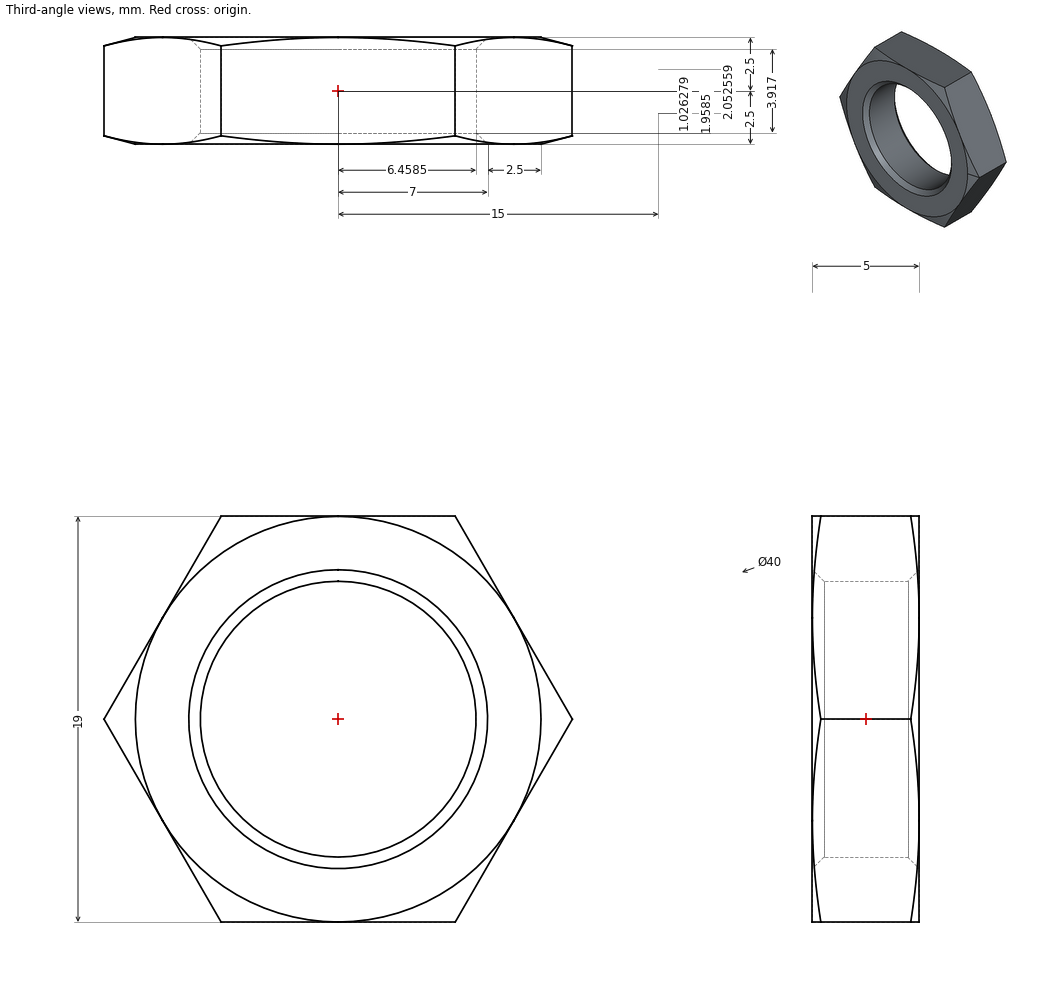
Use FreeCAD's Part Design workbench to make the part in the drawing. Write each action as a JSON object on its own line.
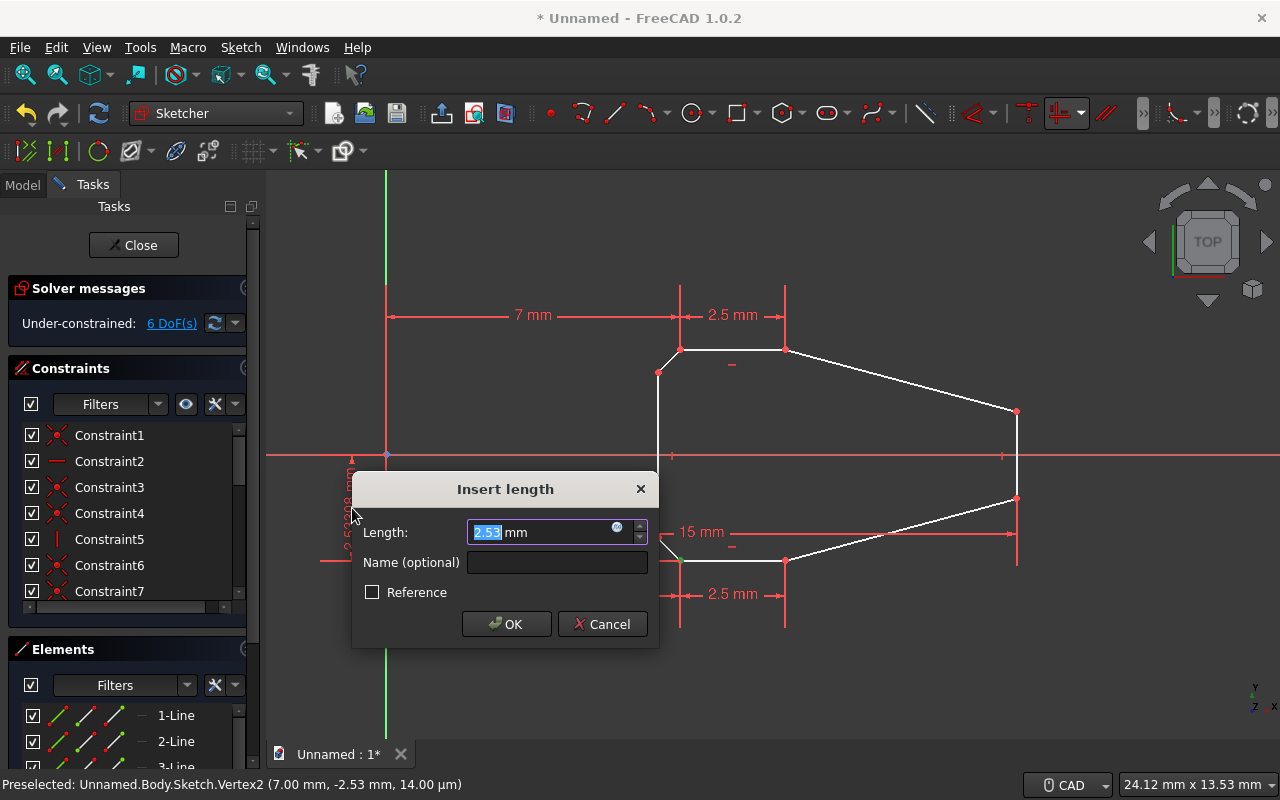
{"action": "type", "text": "2.5"}
{"action": "key", "text": "Return"}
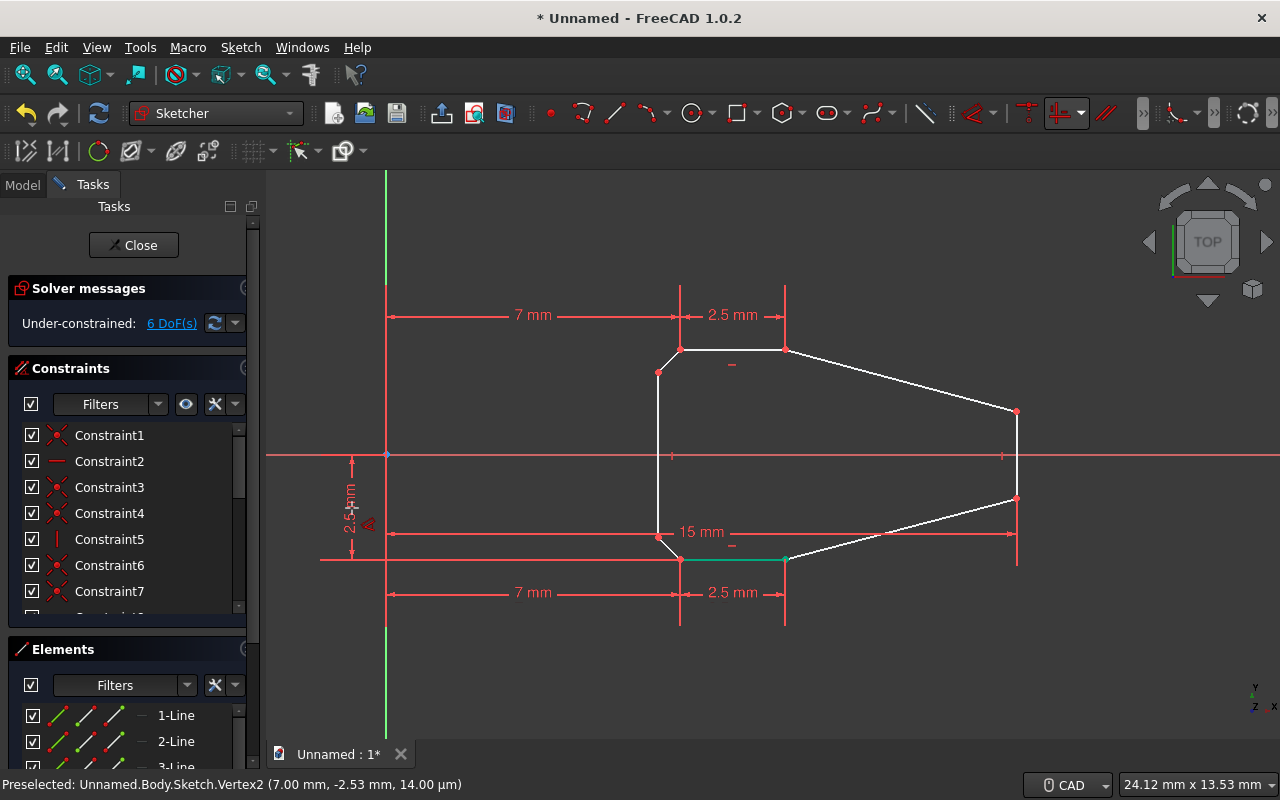
{"action": "left_click", "coordinate": [785, 350]}
{"action": "left_click", "coordinate": [352, 402]}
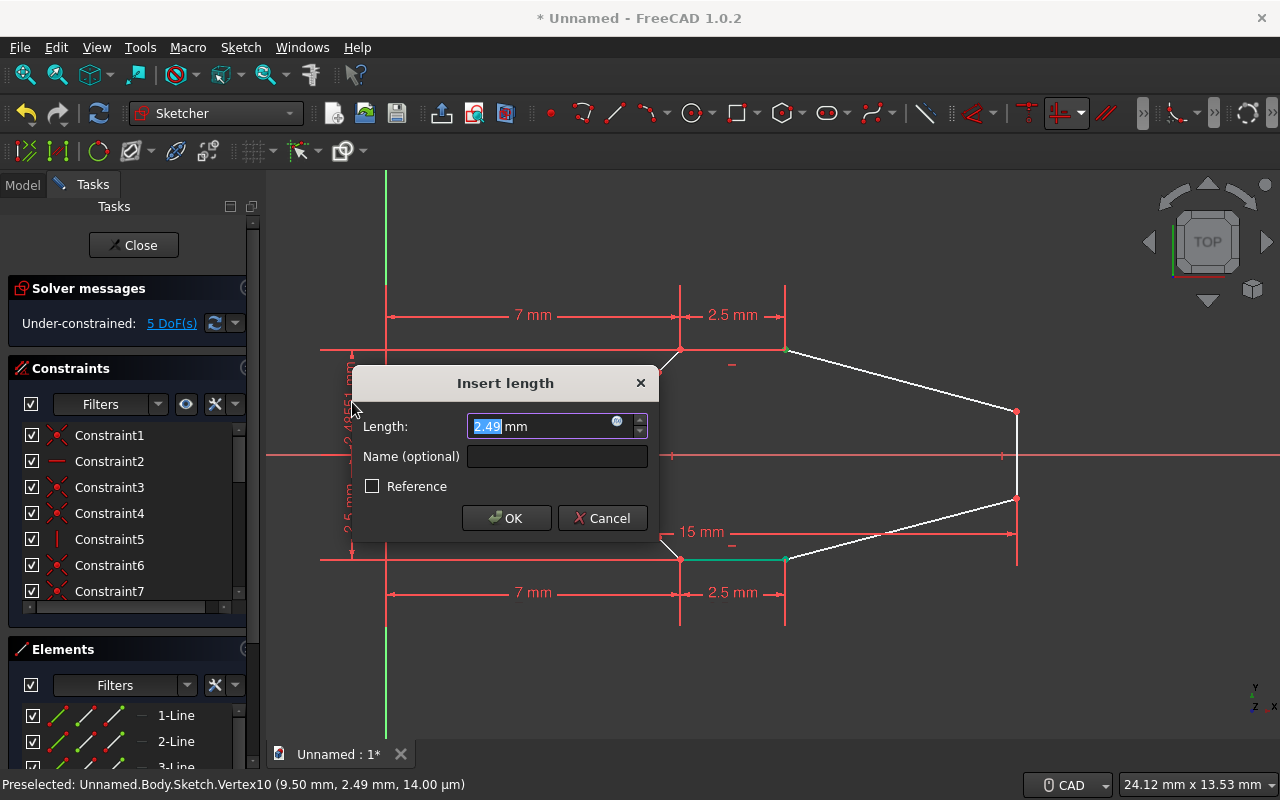
{"action": "type", "text": "2.5"}
{"action": "key", "text": "Return"}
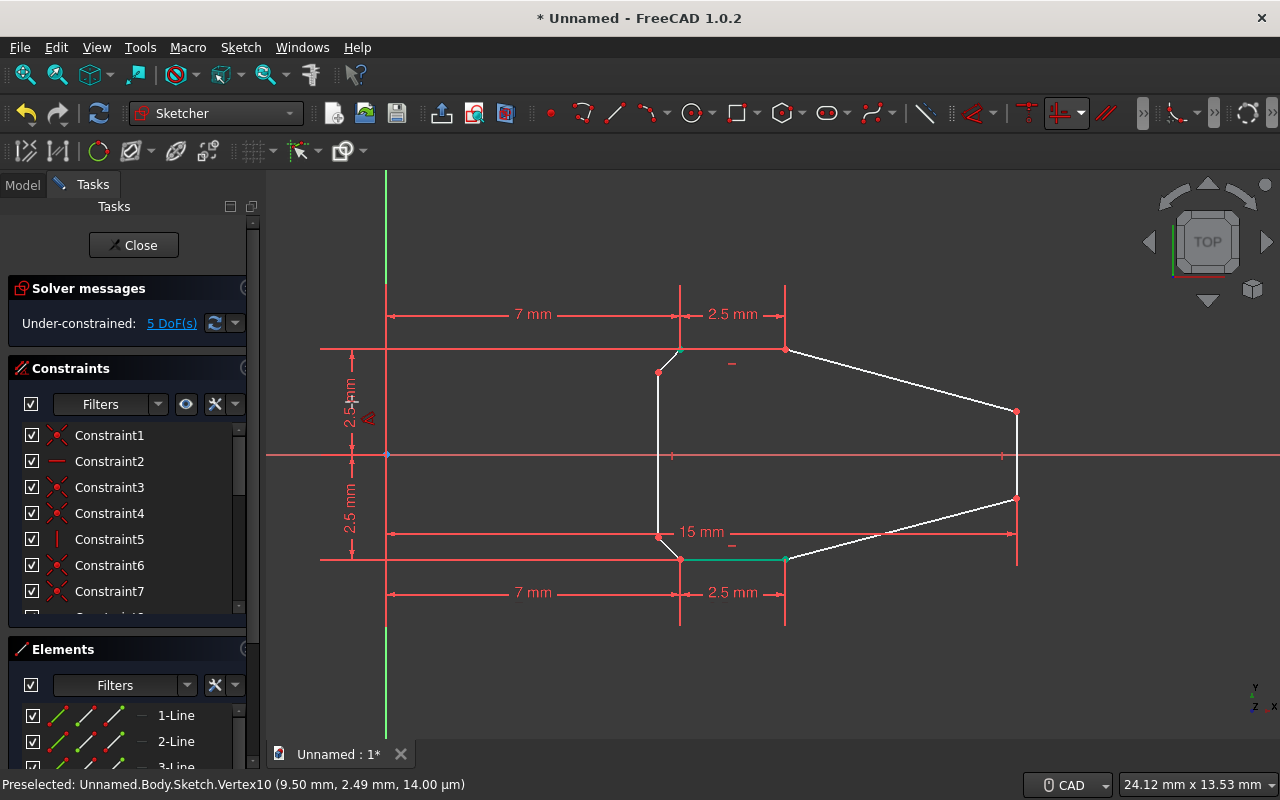
{"action": "left_click", "coordinate": [658, 423]}
{"action": "left_click", "coordinate": [624, 418]}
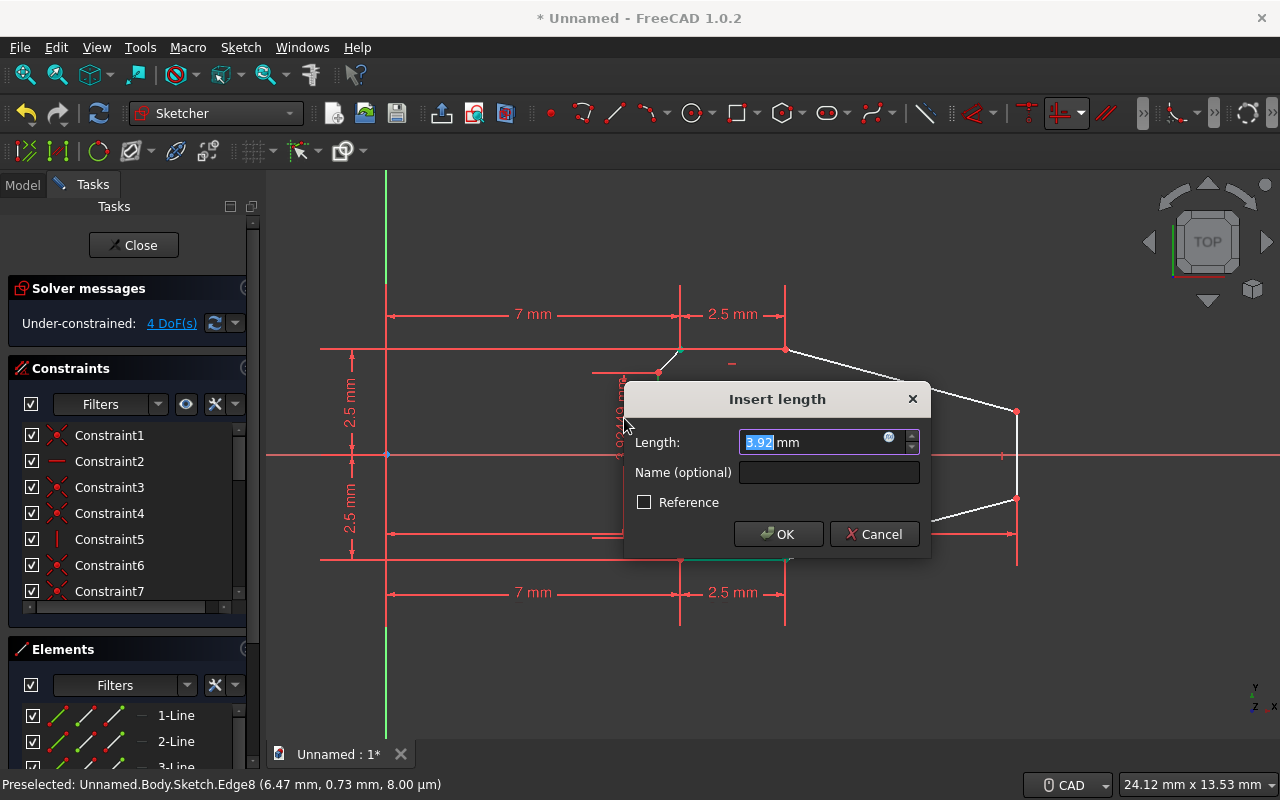
{"action": "type", "text": "3.917"}
{"action": "key", "text": "Return"}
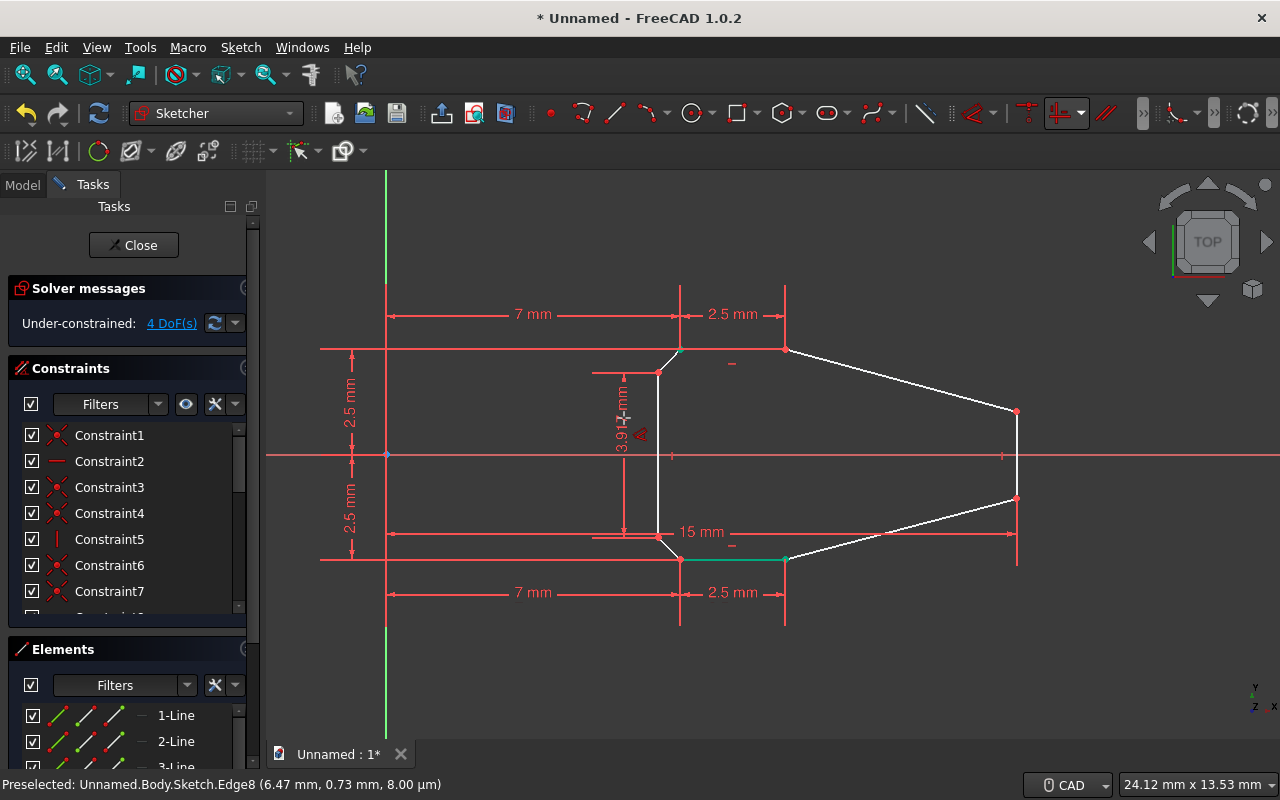
{"action": "left_click", "coordinate": [658, 538]}
{"action": "left_click", "coordinate": [522, 572]}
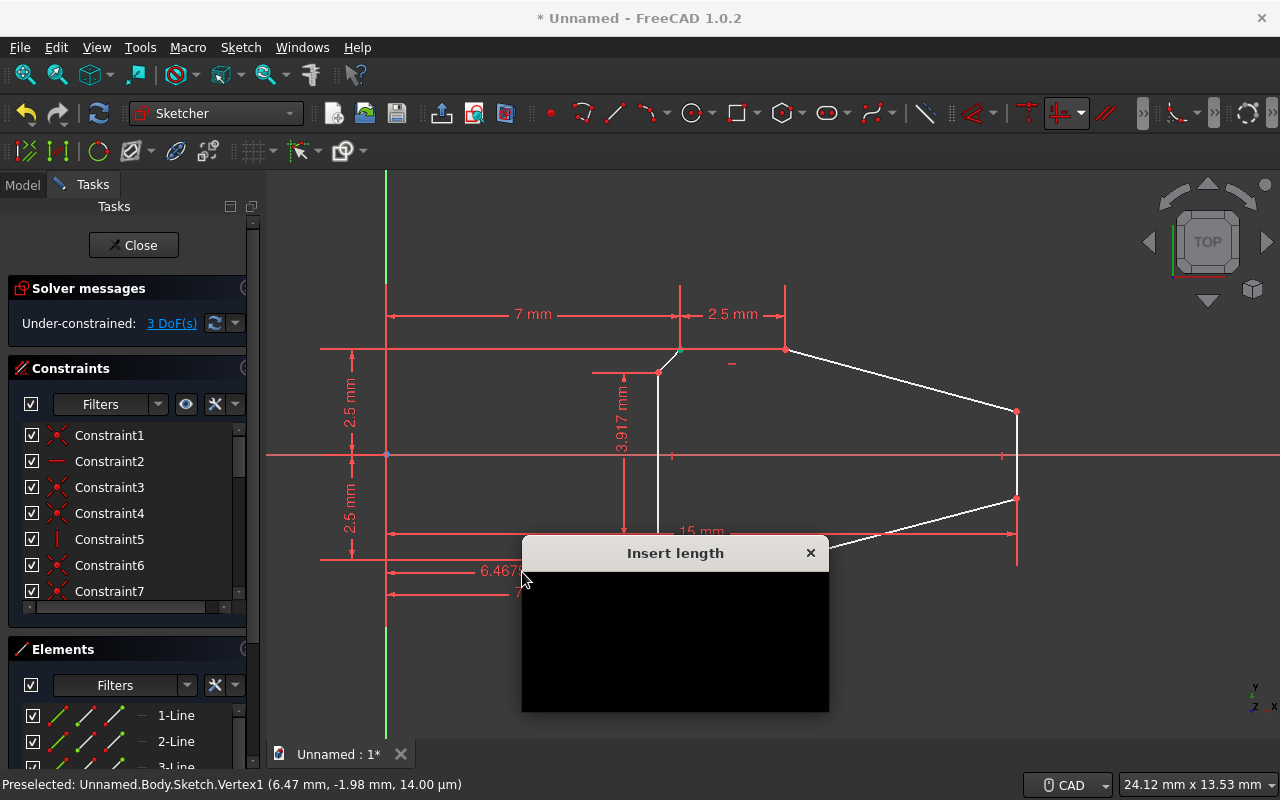
{"action": "type", "text": "6.4585"}
{"action": "key", "text": "Return"}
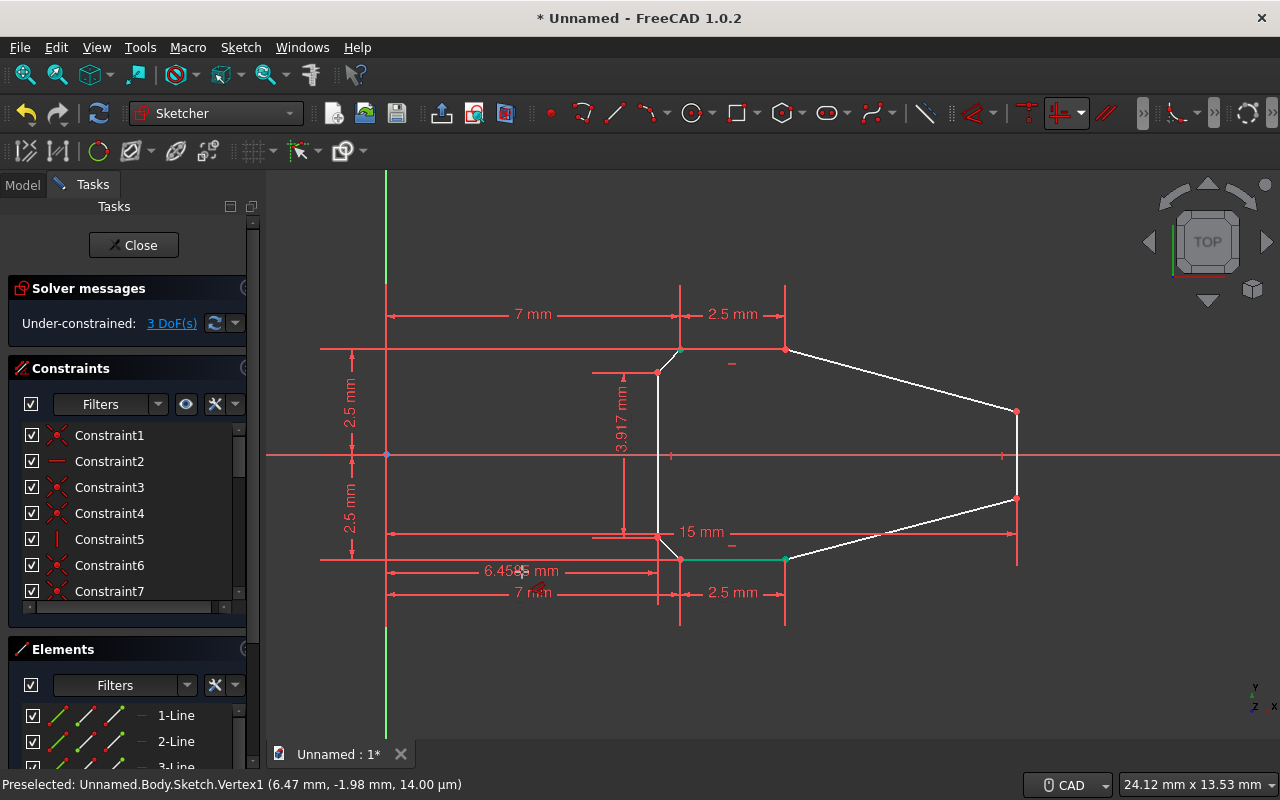
{"action": "left_click", "coordinate": [658, 538]}
{"action": "left_click", "coordinate": [352, 477]}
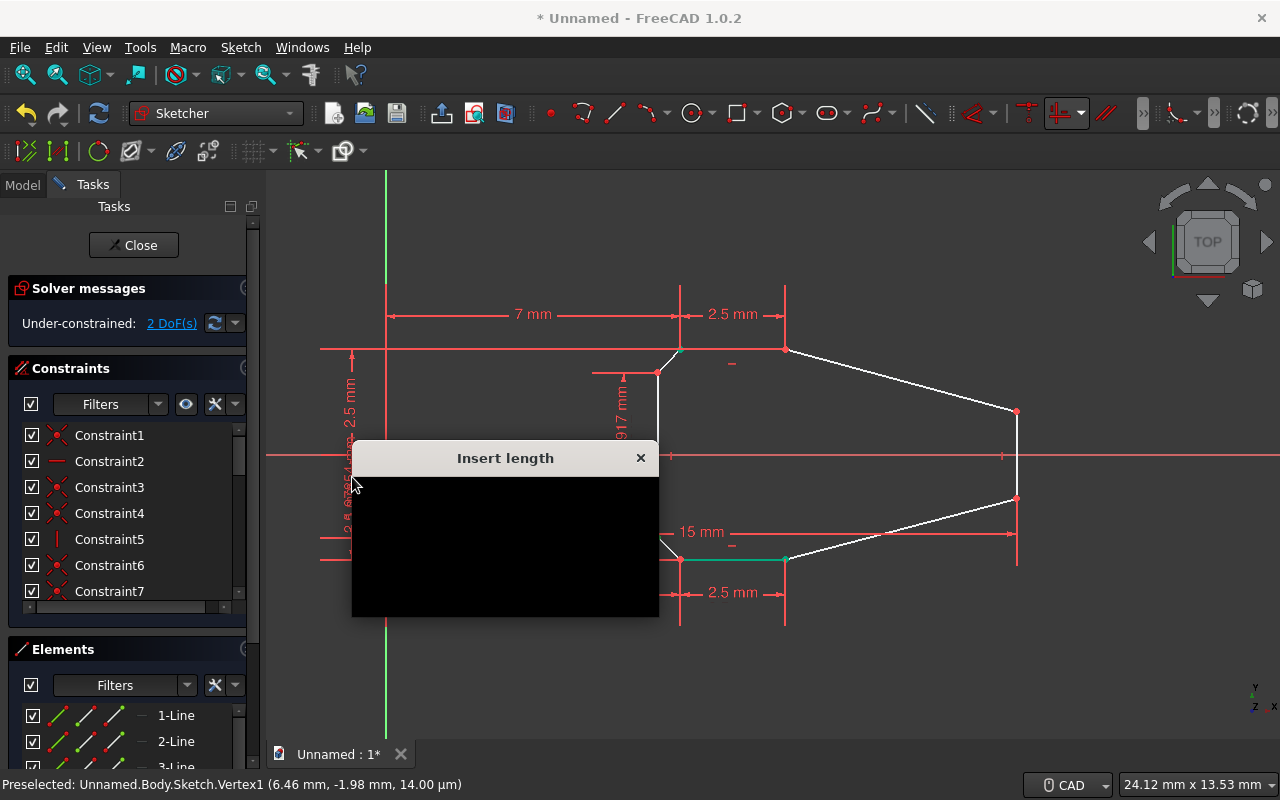
{"action": "type", "text": "1.9585"}
{"action": "key", "text": "Return"}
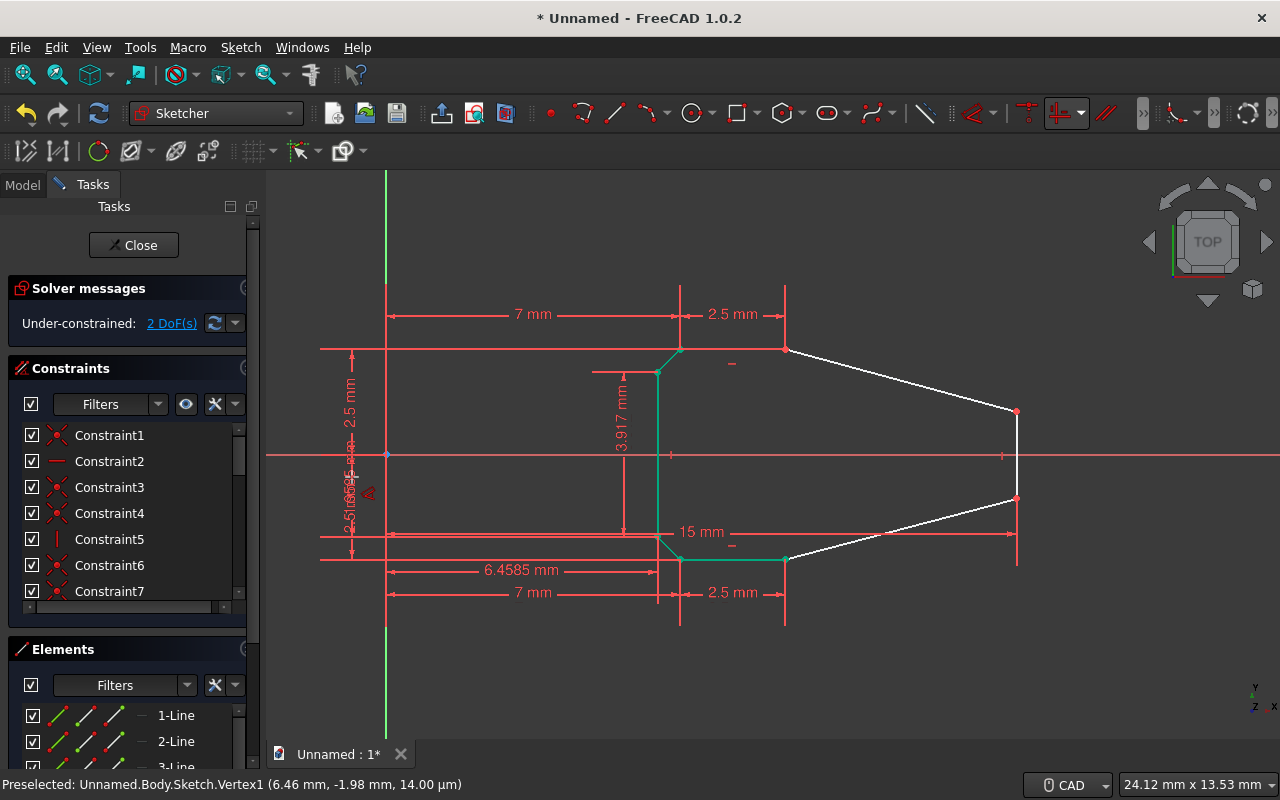
{"action": "left_click", "coordinate": [1017, 473]}
{"action": "left_click", "coordinate": [1051, 435]}